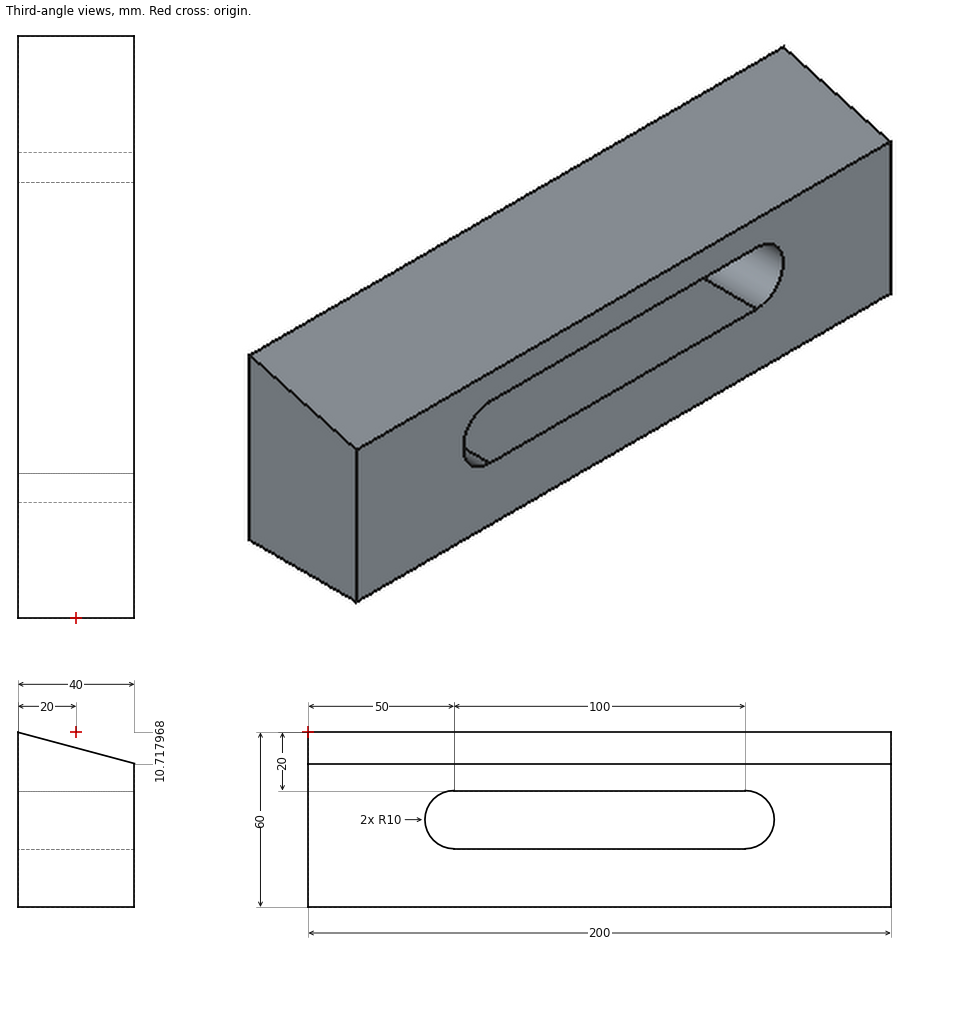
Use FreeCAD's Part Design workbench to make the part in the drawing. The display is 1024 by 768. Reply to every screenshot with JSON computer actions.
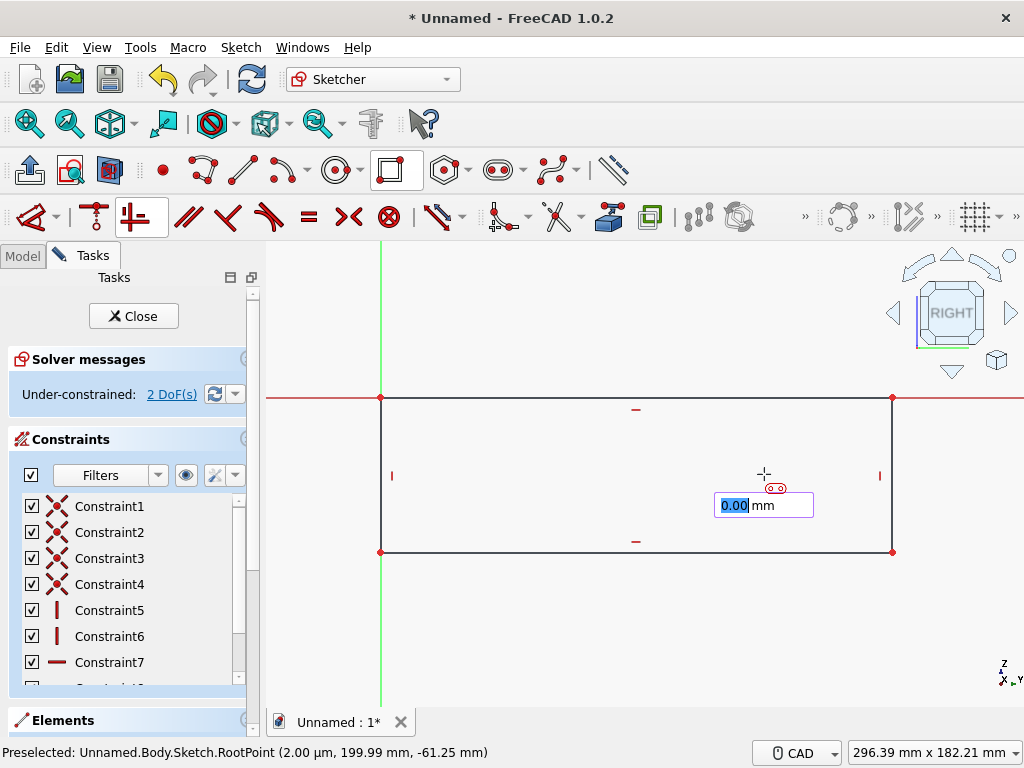
{"action": "left_click", "coordinate": [637, 449]}
{"action": "key", "text": "Escape"}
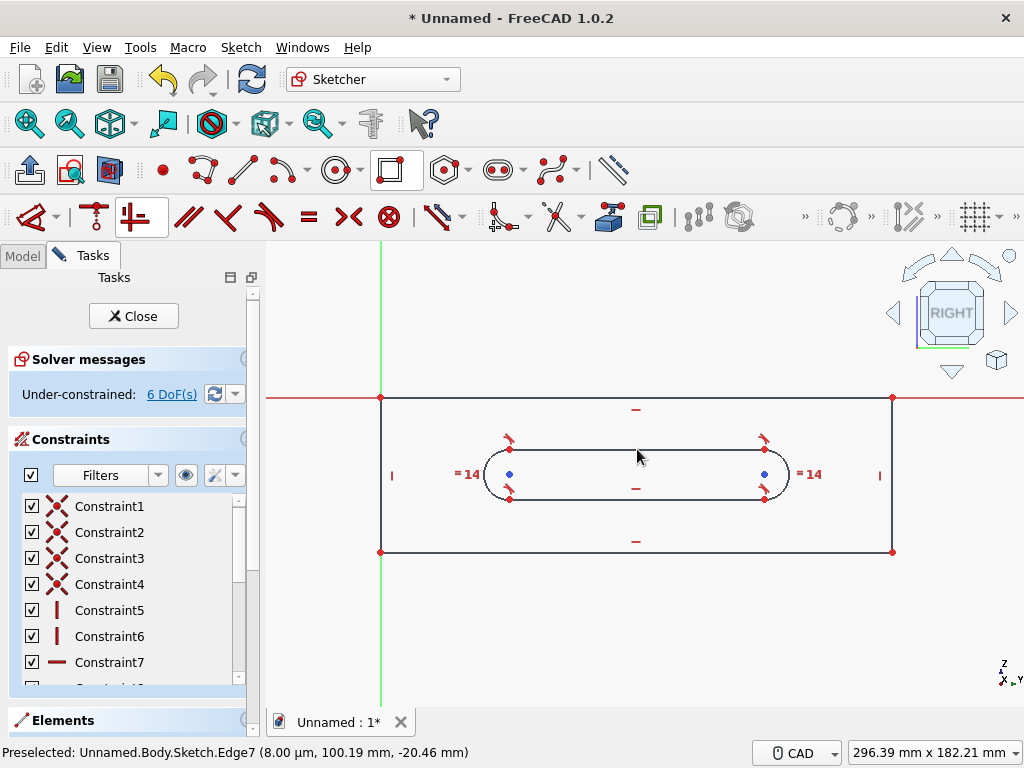
{"action": "left_click", "coordinate": [32, 218]}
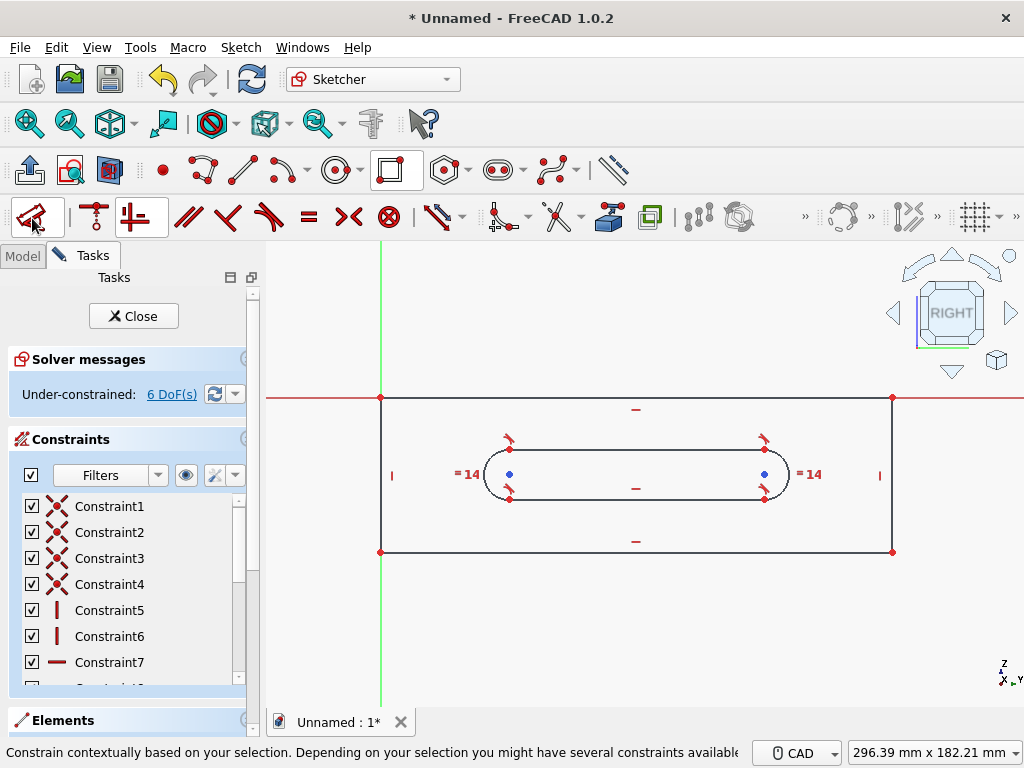
{"action": "scroll", "coordinate": [489, 460], "scroll_direction": "up", "scroll_amount": 3}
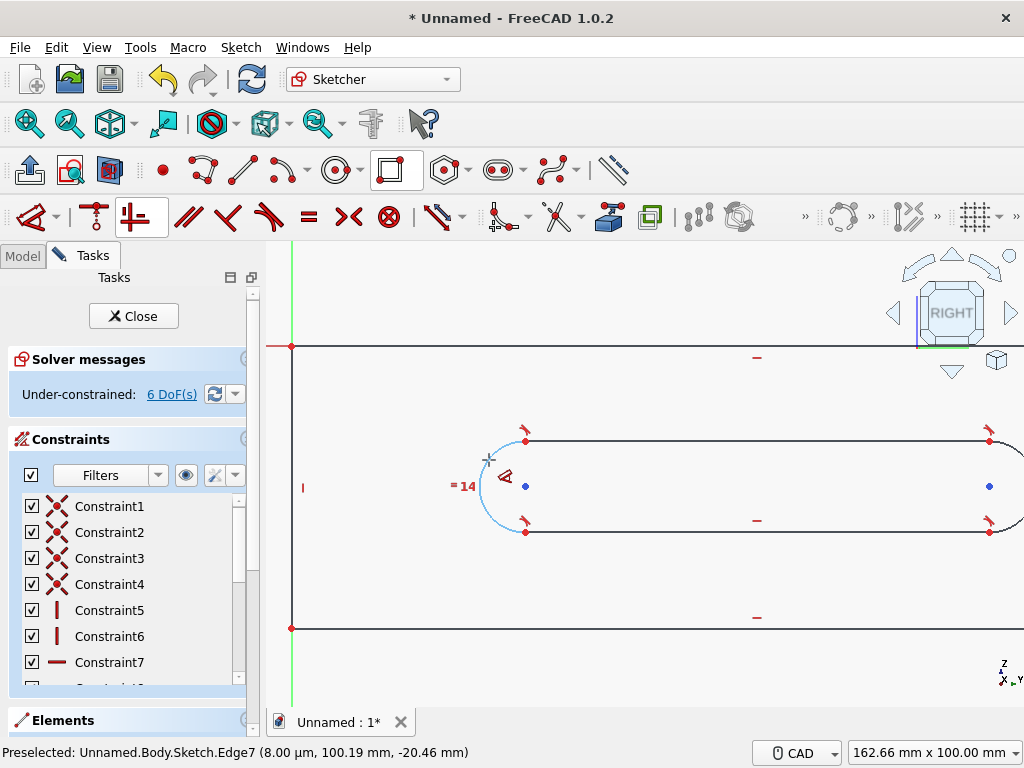
{"action": "left_click", "coordinate": [488, 460]}
{"action": "left_click", "coordinate": [462, 441]}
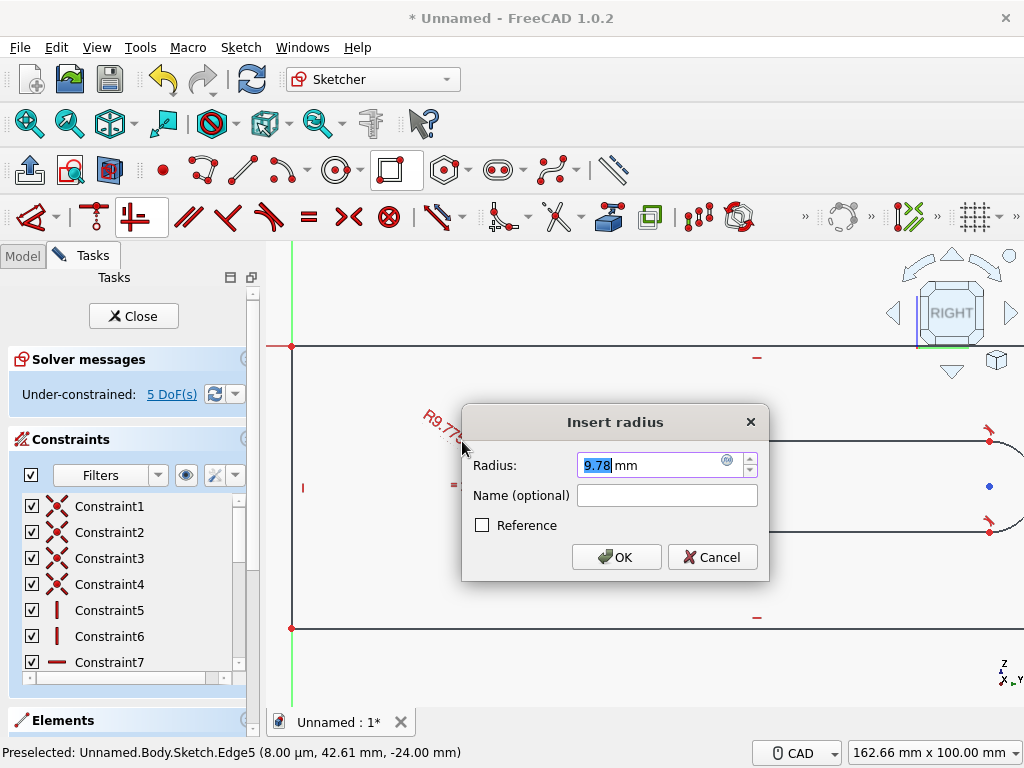
{"action": "type", "text": "10"}
{"action": "key", "text": "Return"}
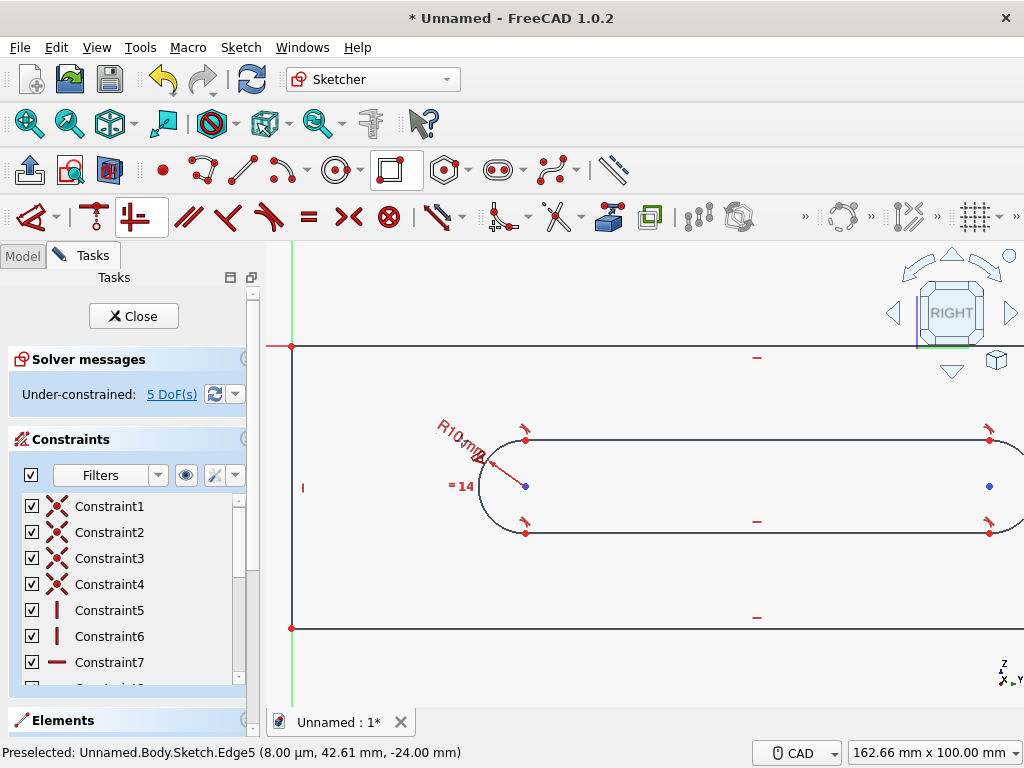
{"action": "scroll", "coordinate": [429, 464], "scroll_direction": "down", "scroll_amount": 4}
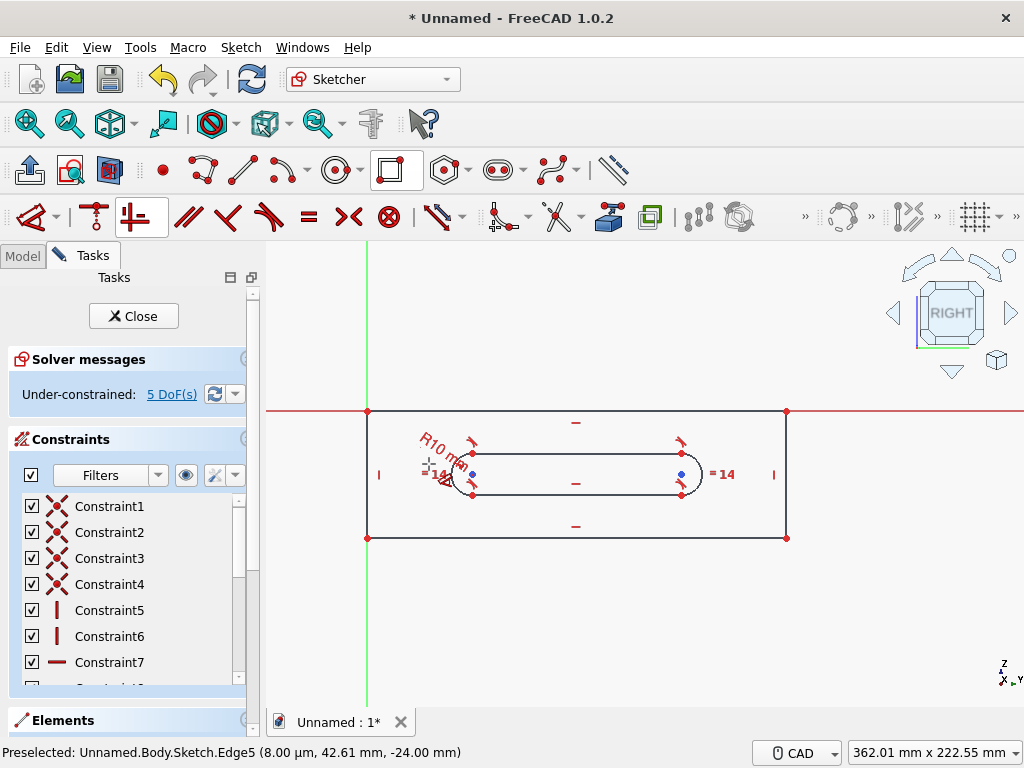
{"action": "left_click", "coordinate": [367, 449]}
{"action": "left_click", "coordinate": [333, 475]}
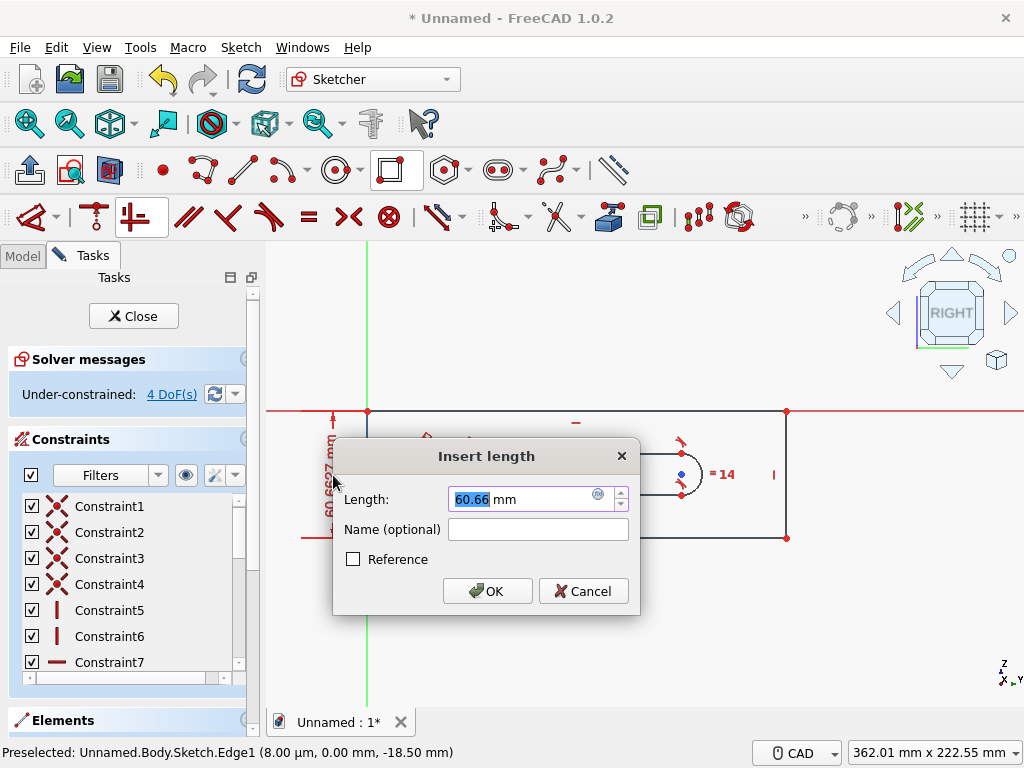
{"action": "type", "text": "60"}
{"action": "key", "text": "Return"}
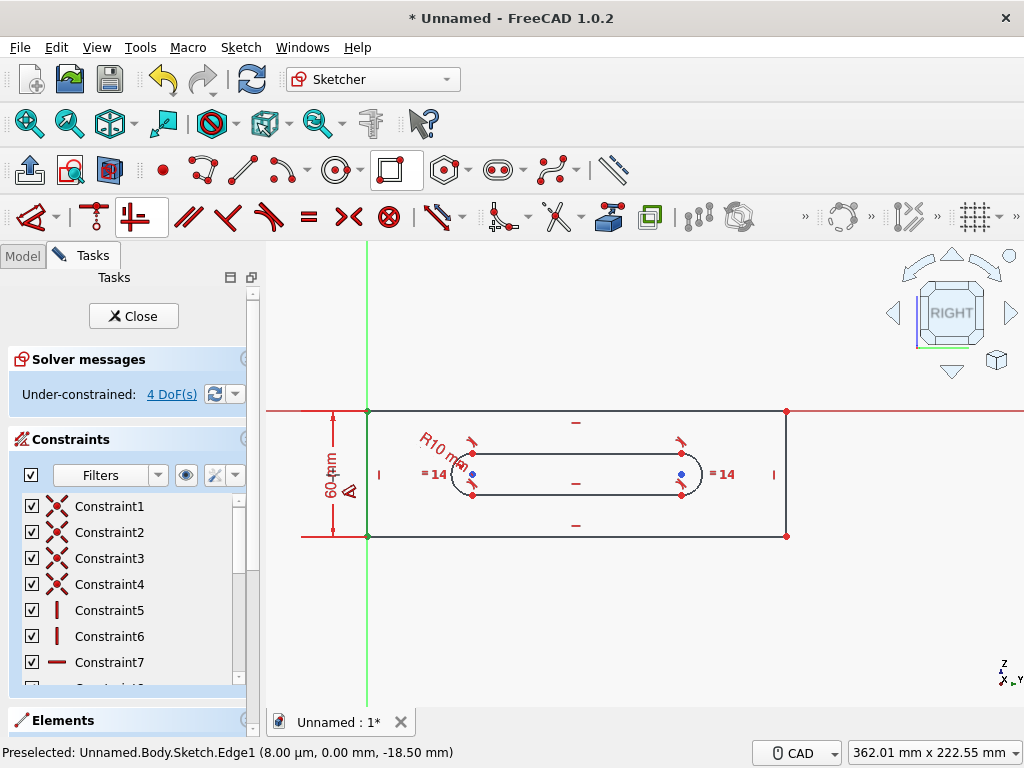
{"action": "left_click", "coordinate": [493, 537]}
{"action": "left_click", "coordinate": [577, 571]}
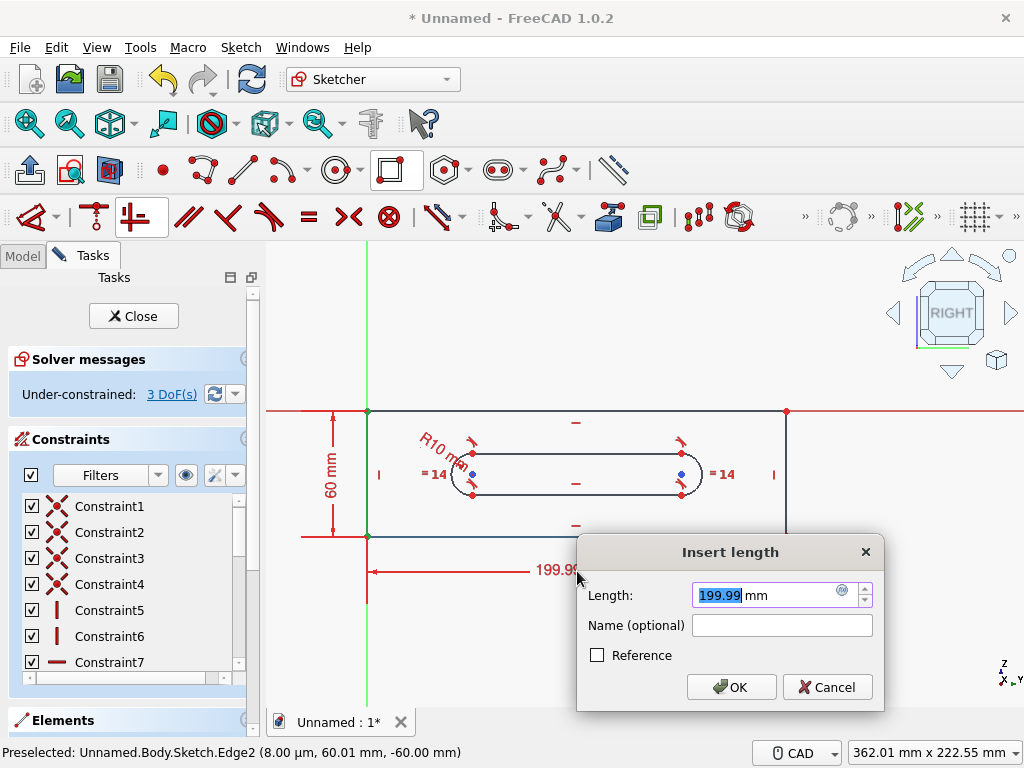
{"action": "type", "text": "200"}
{"action": "key", "text": "Return"}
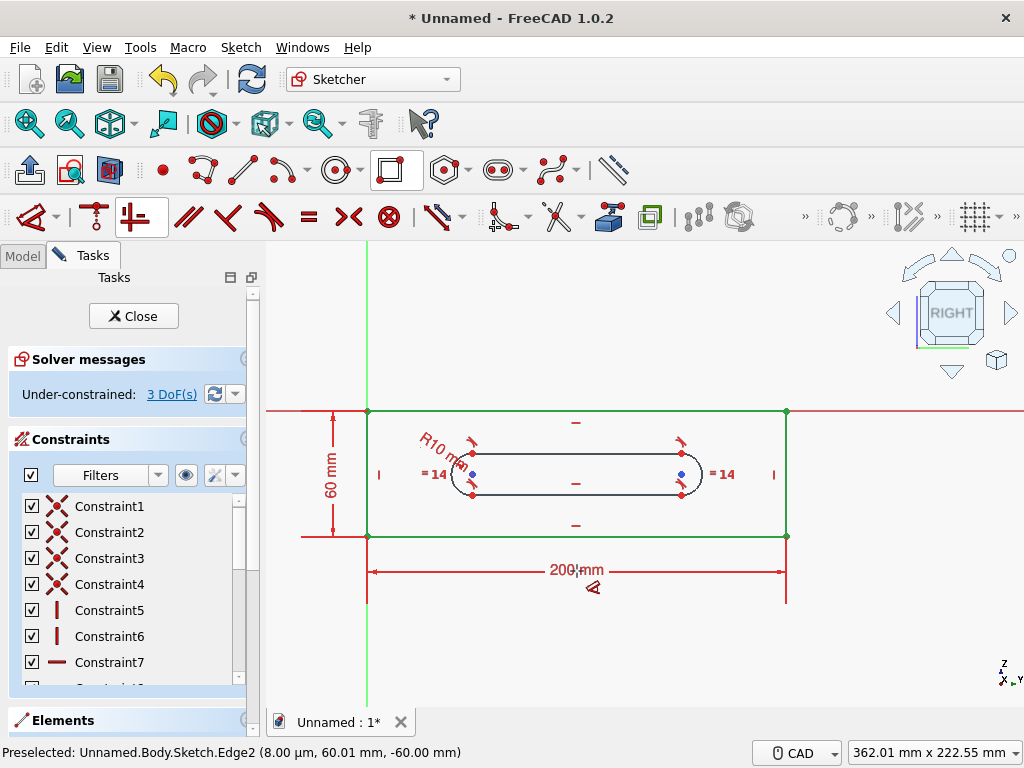
{"action": "left_click", "coordinate": [535, 454]}
{"action": "left_click", "coordinate": [577, 396]}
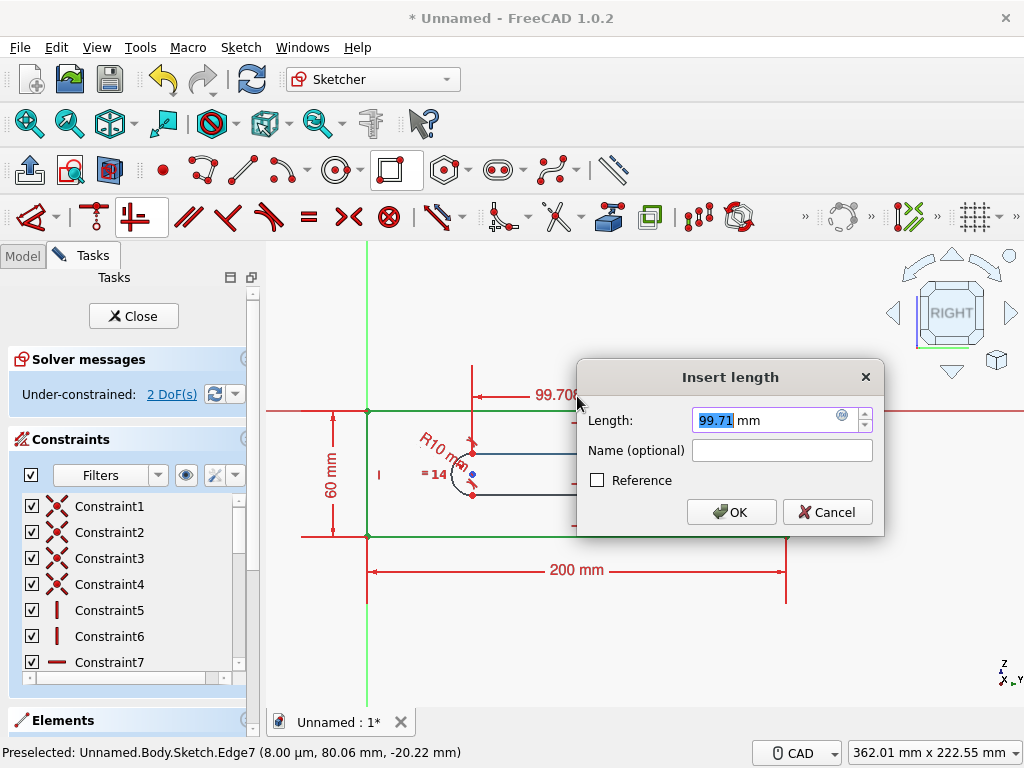
{"action": "type", "text": "100"}
{"action": "key", "text": "Return"}